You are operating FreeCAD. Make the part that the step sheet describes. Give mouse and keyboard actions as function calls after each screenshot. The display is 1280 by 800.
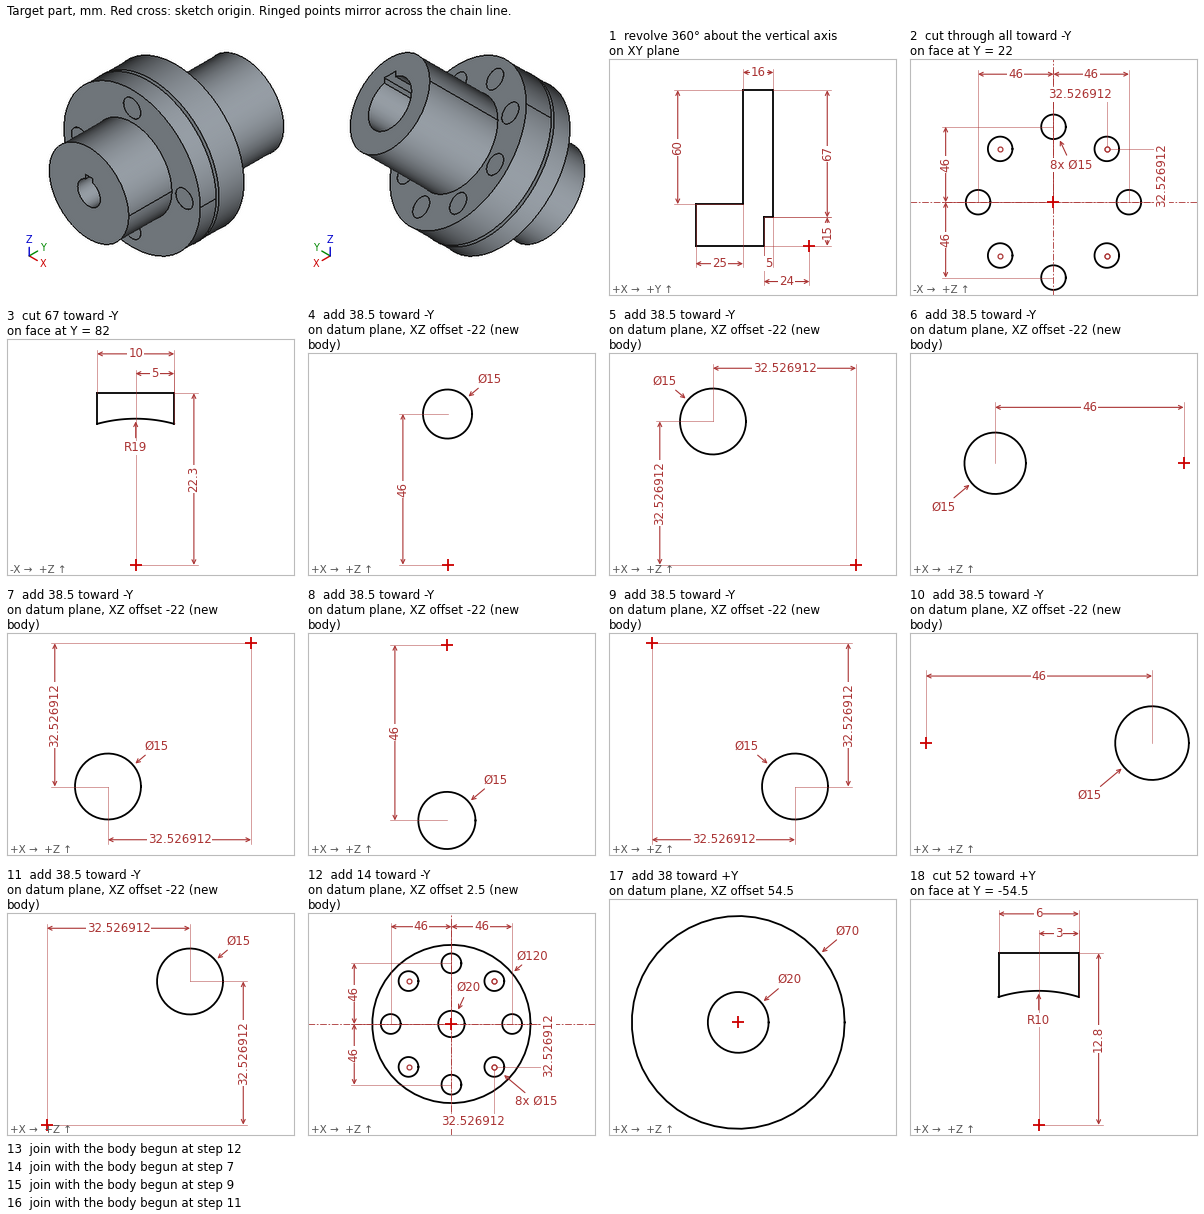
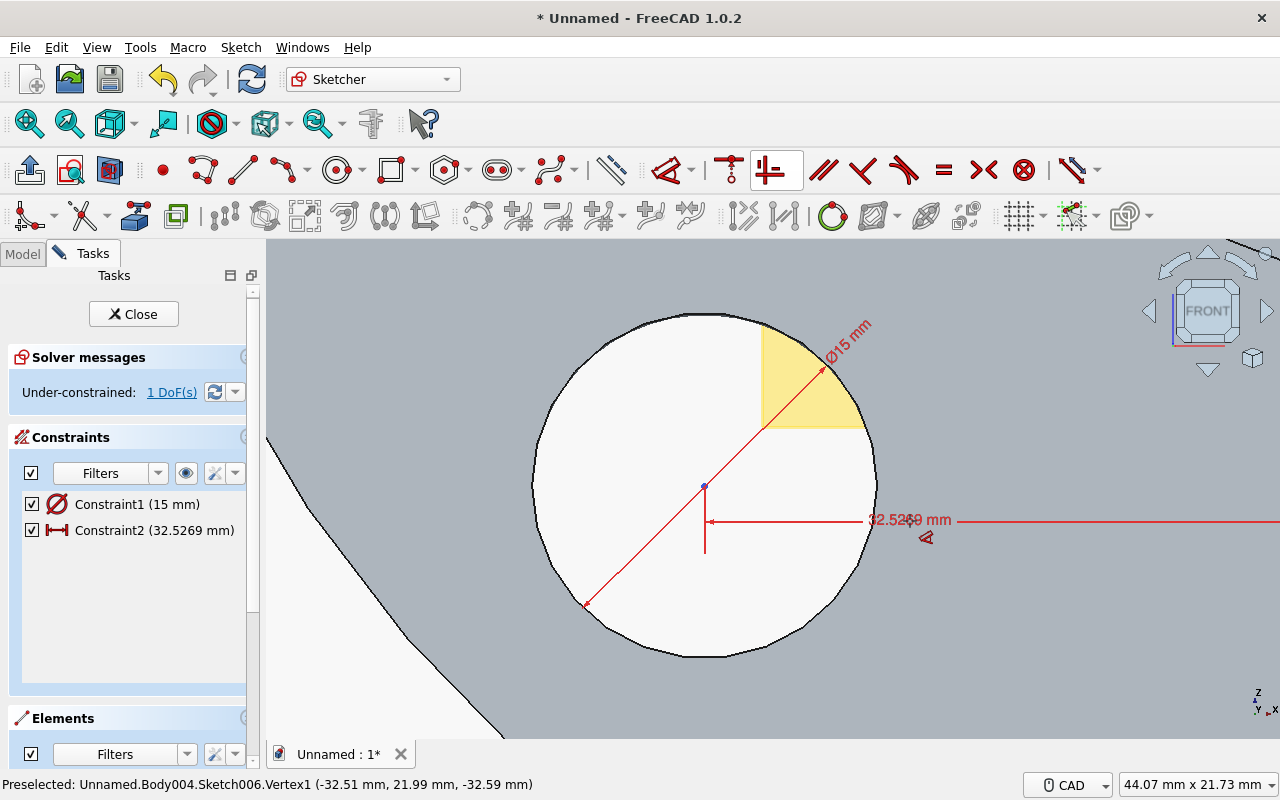
click(705, 487)
click(671, 377)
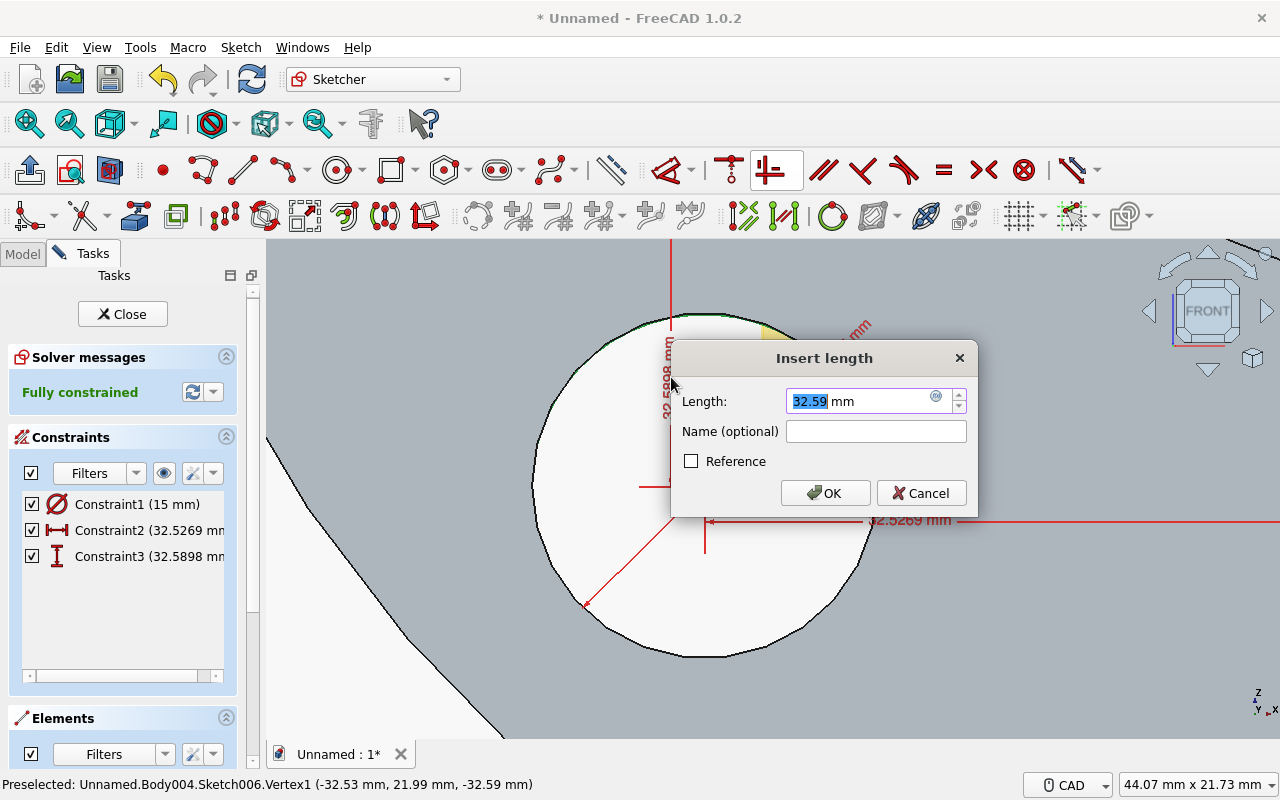
text(32.526912)
key(Return)
key(Escape)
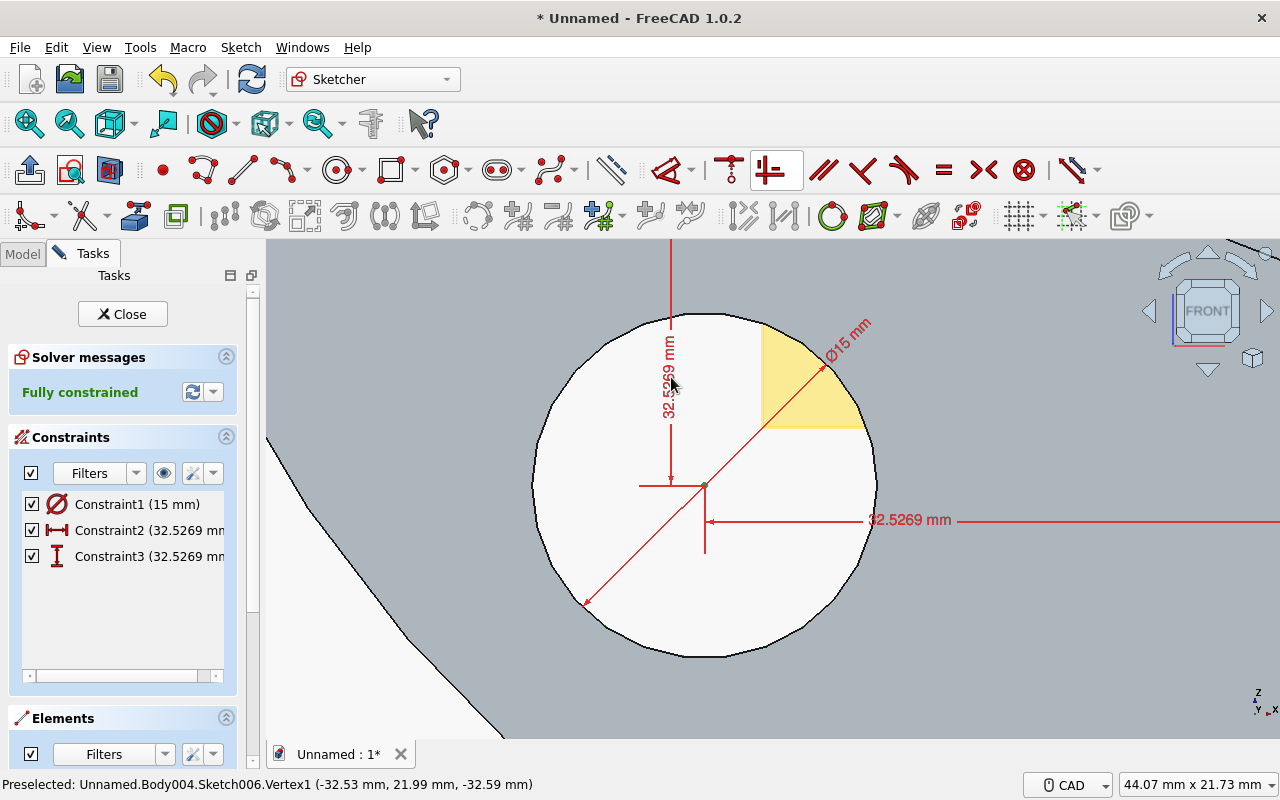
click(123, 314)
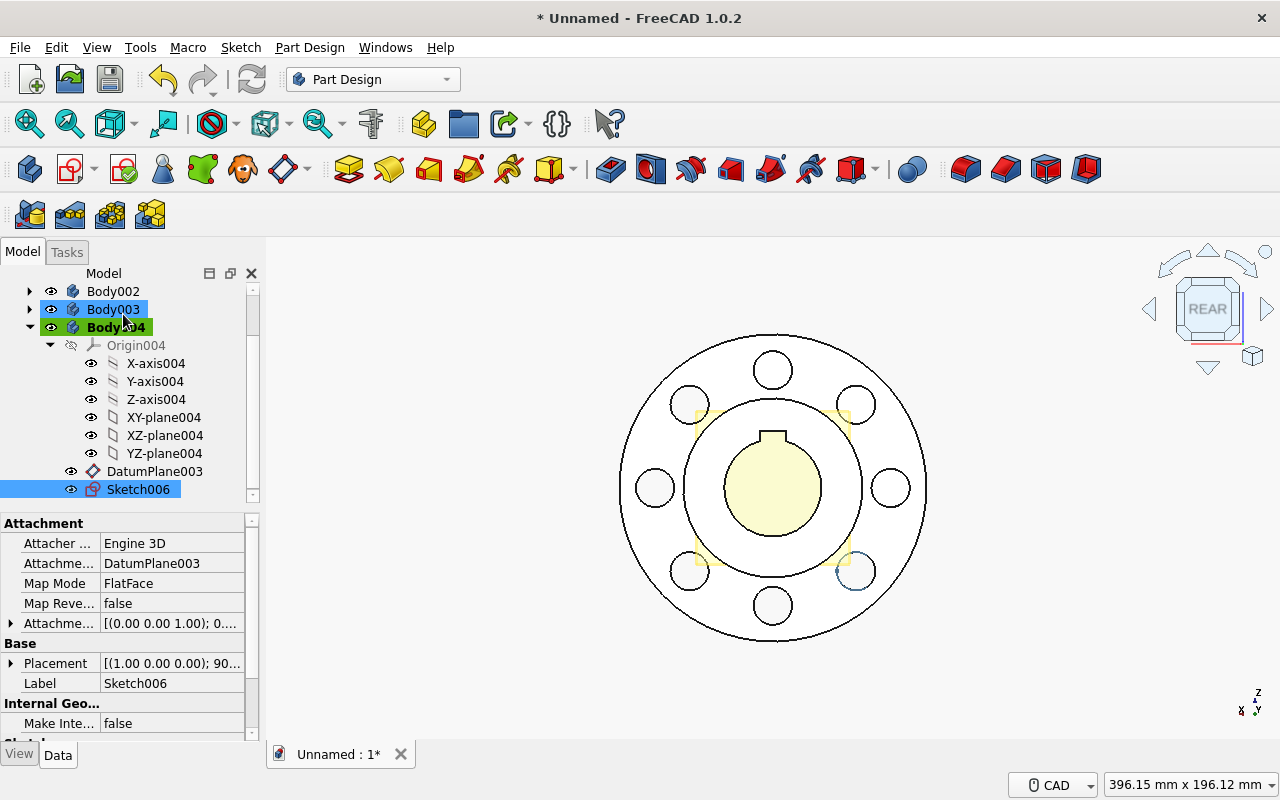
click(350, 170)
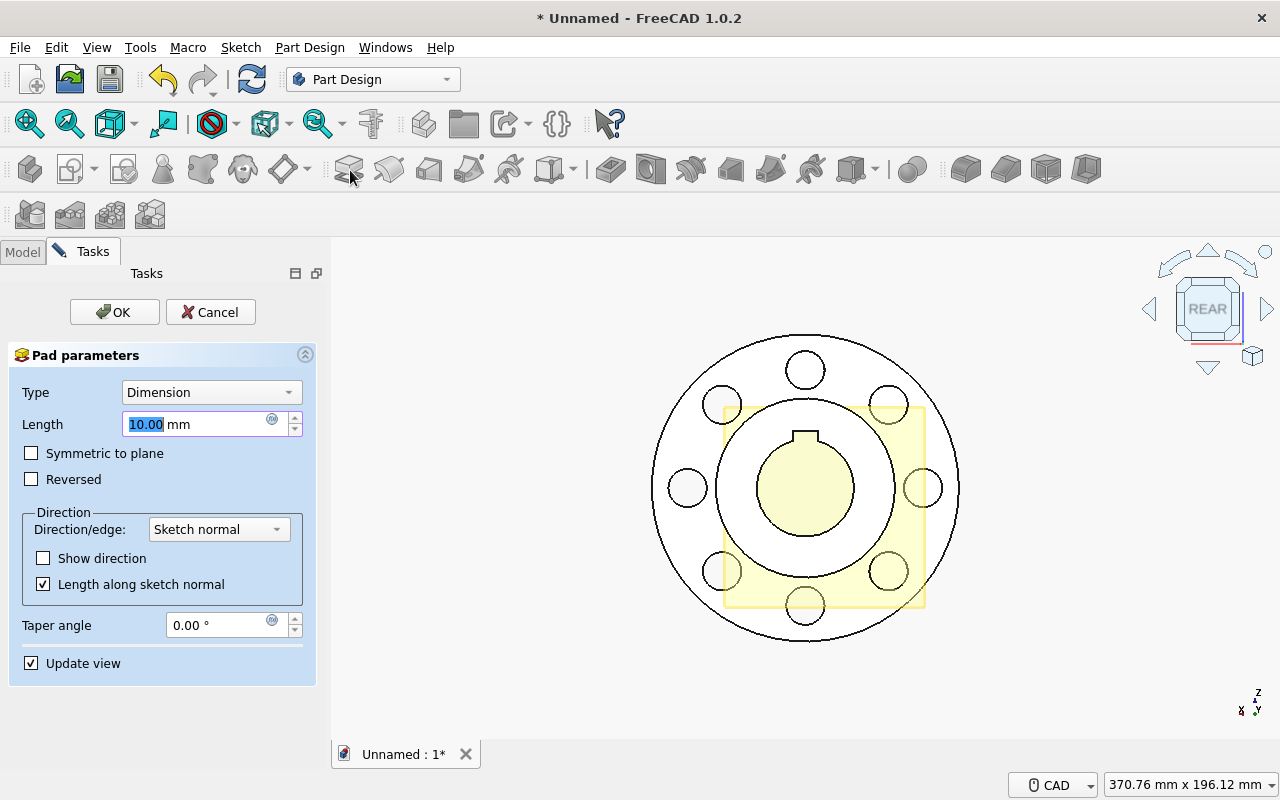
text(38.5)
key(Tab)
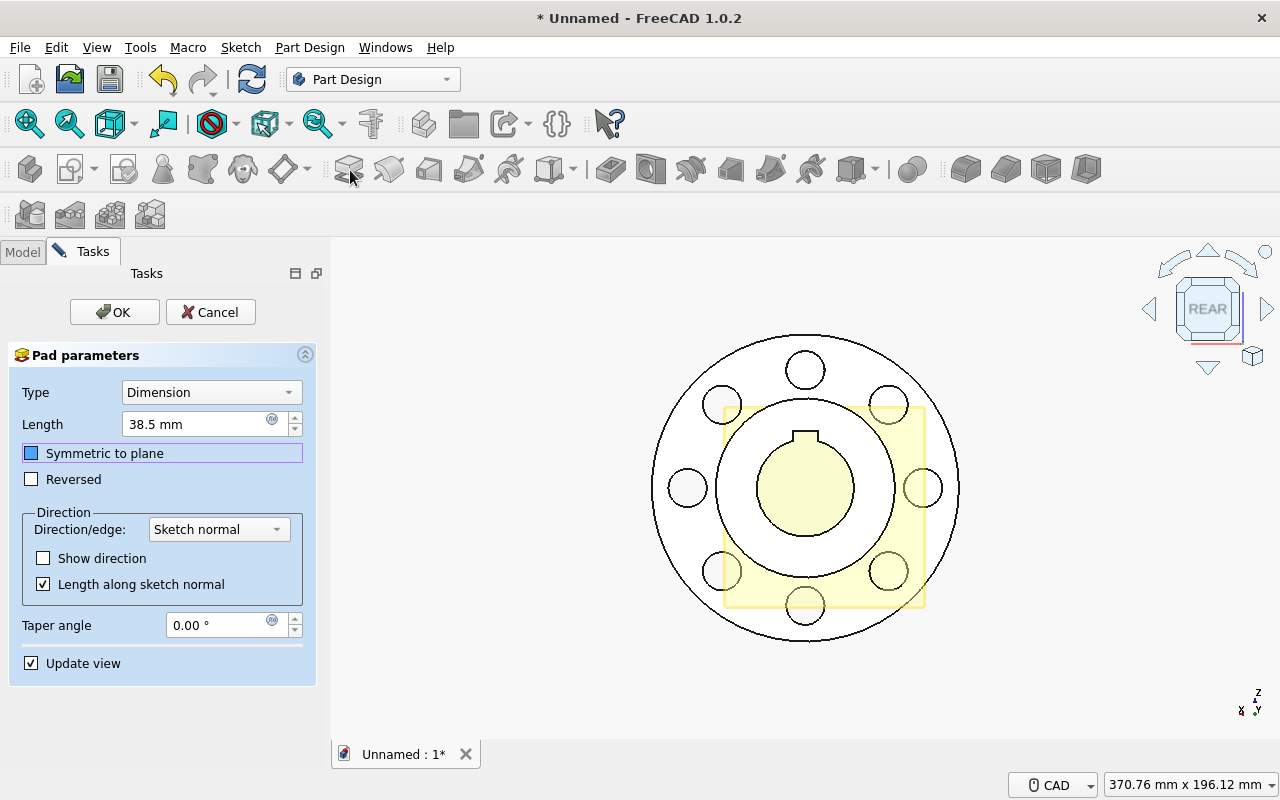
click(115, 312)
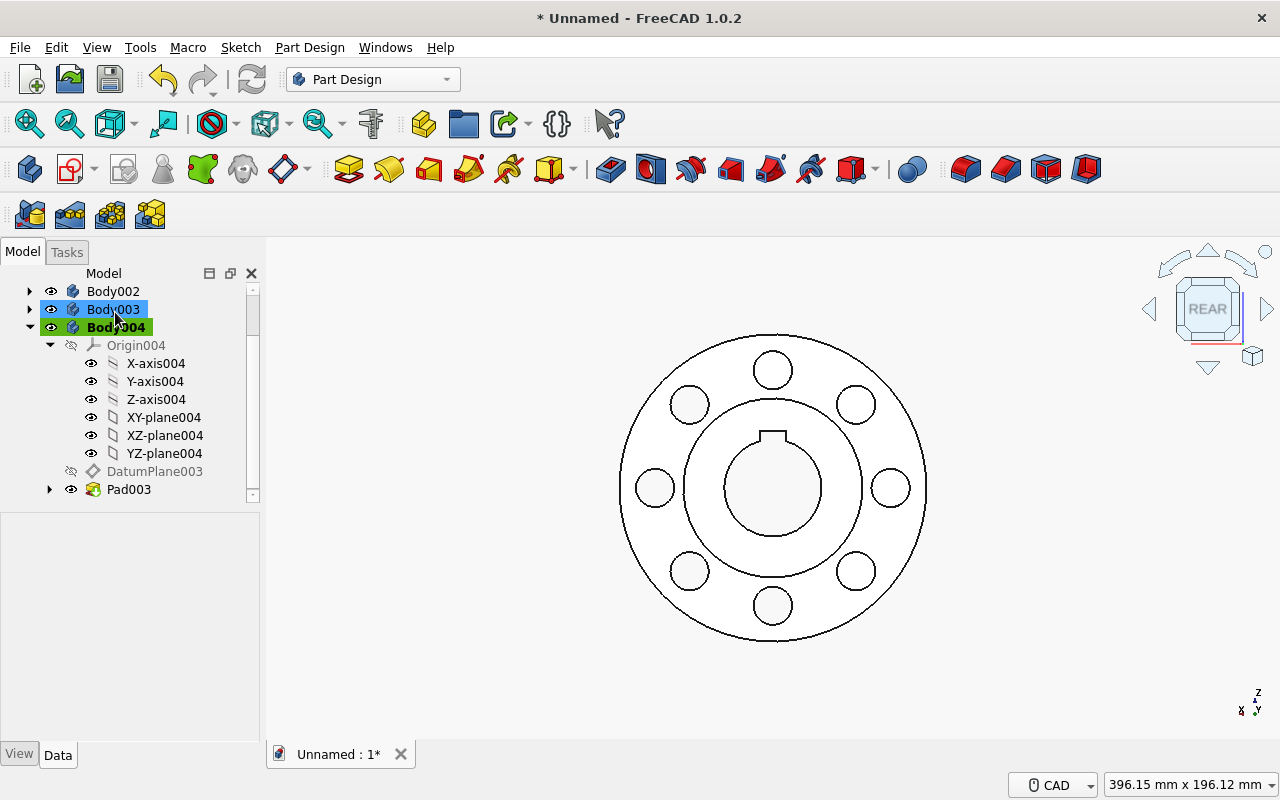
click(30, 124)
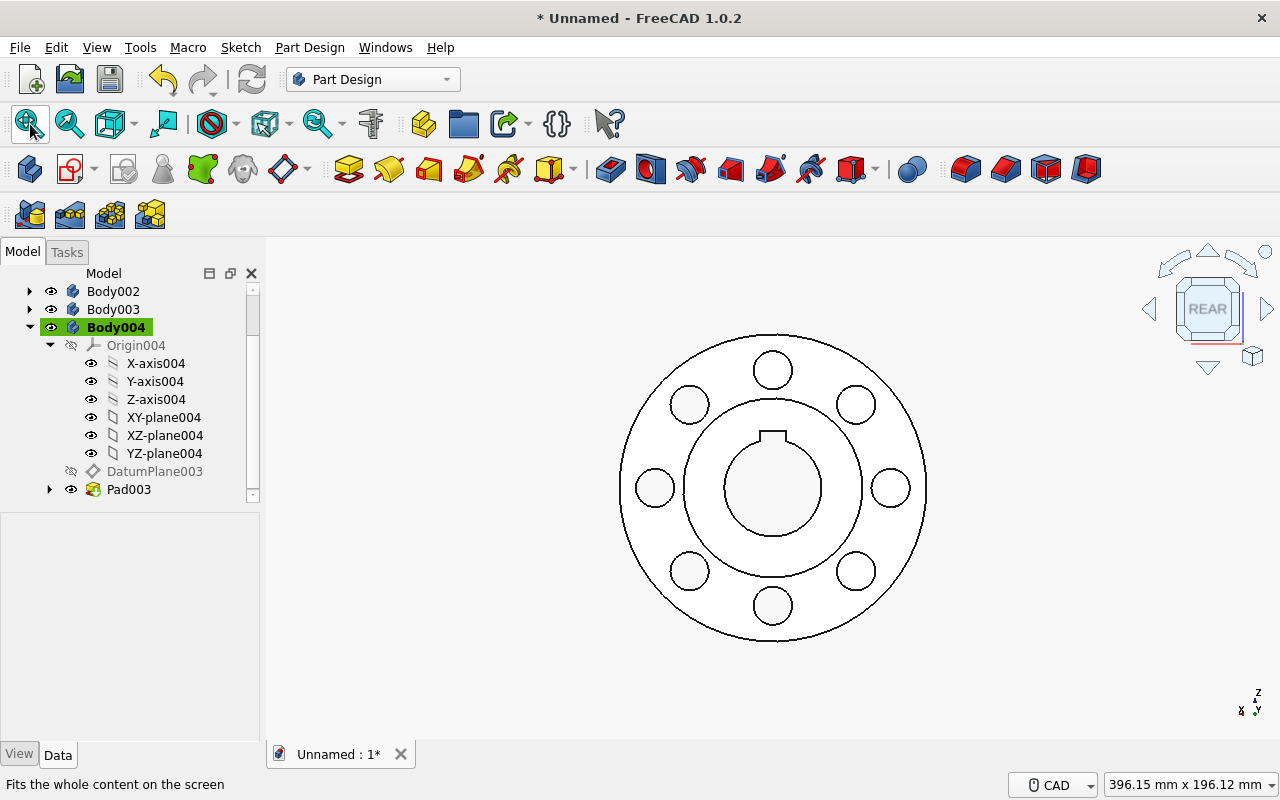
click(30, 170)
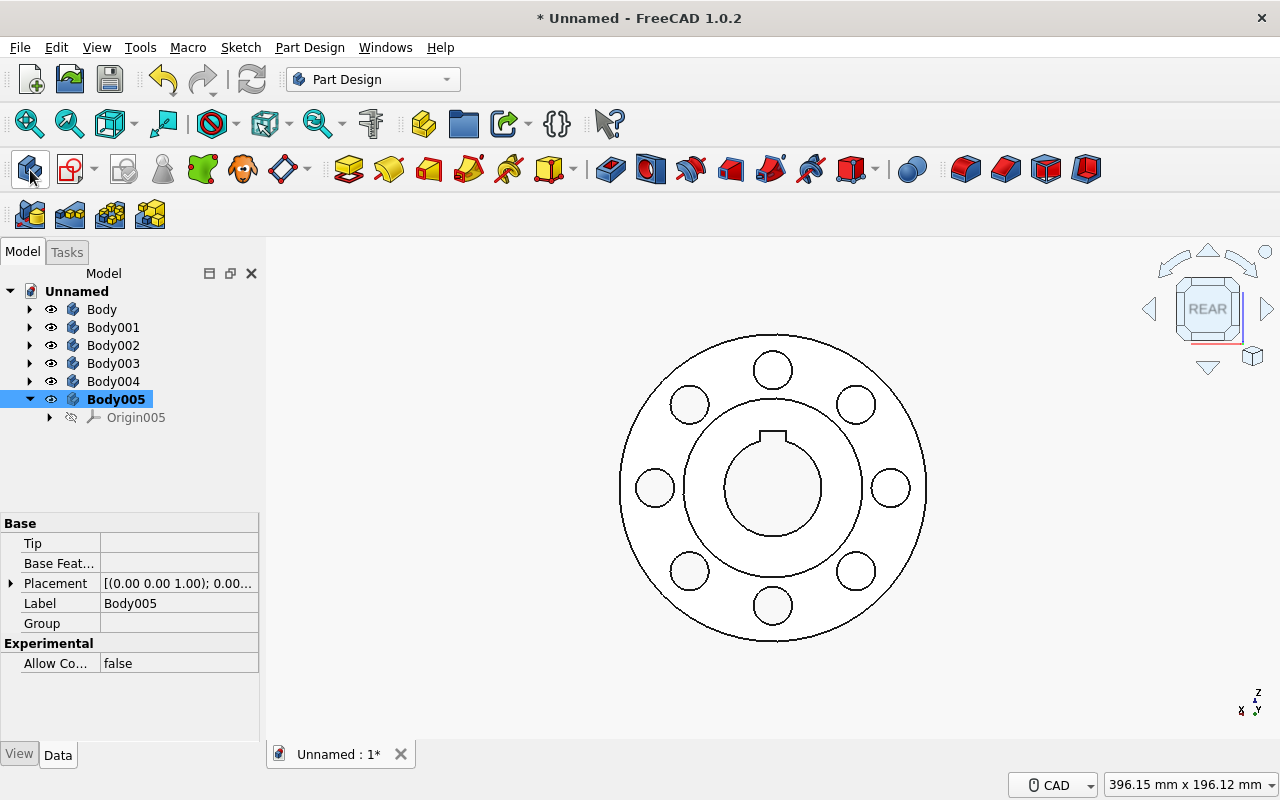
click(50, 417)